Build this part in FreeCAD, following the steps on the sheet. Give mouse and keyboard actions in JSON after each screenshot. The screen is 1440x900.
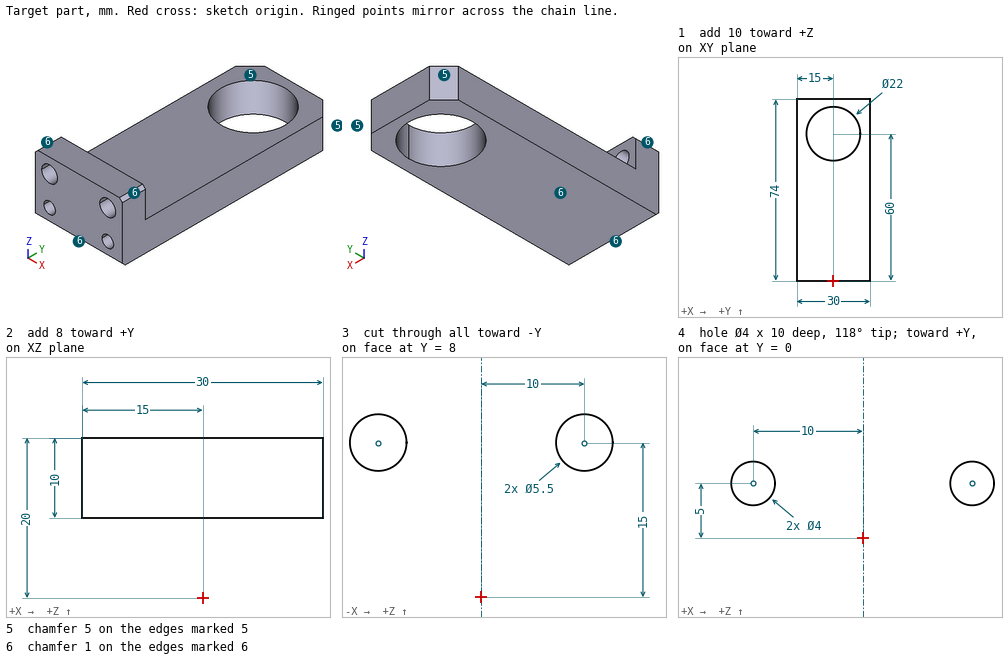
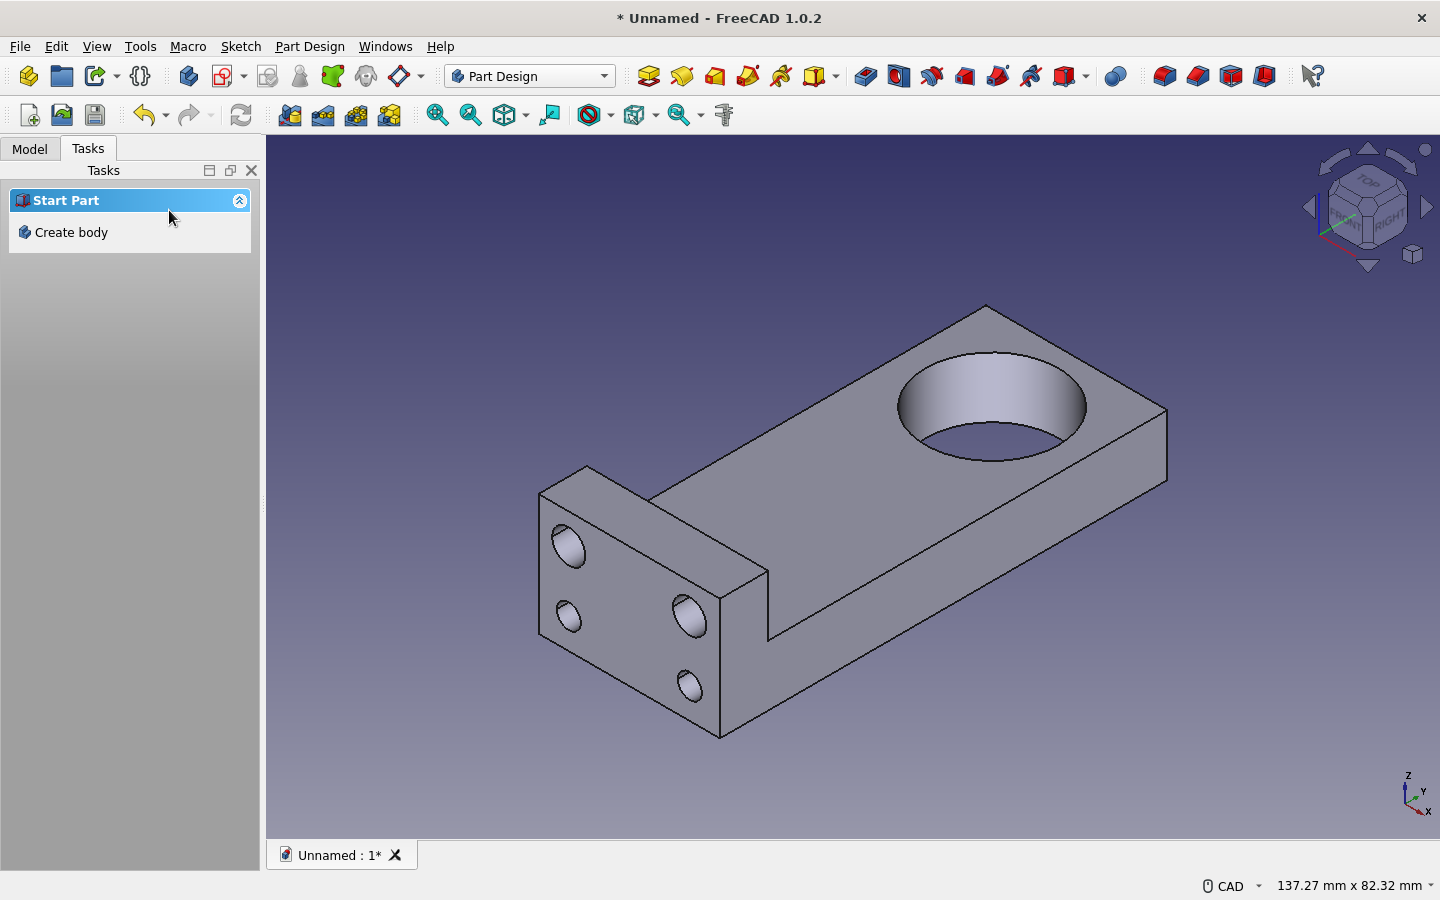
{"action": "key", "text": "1"}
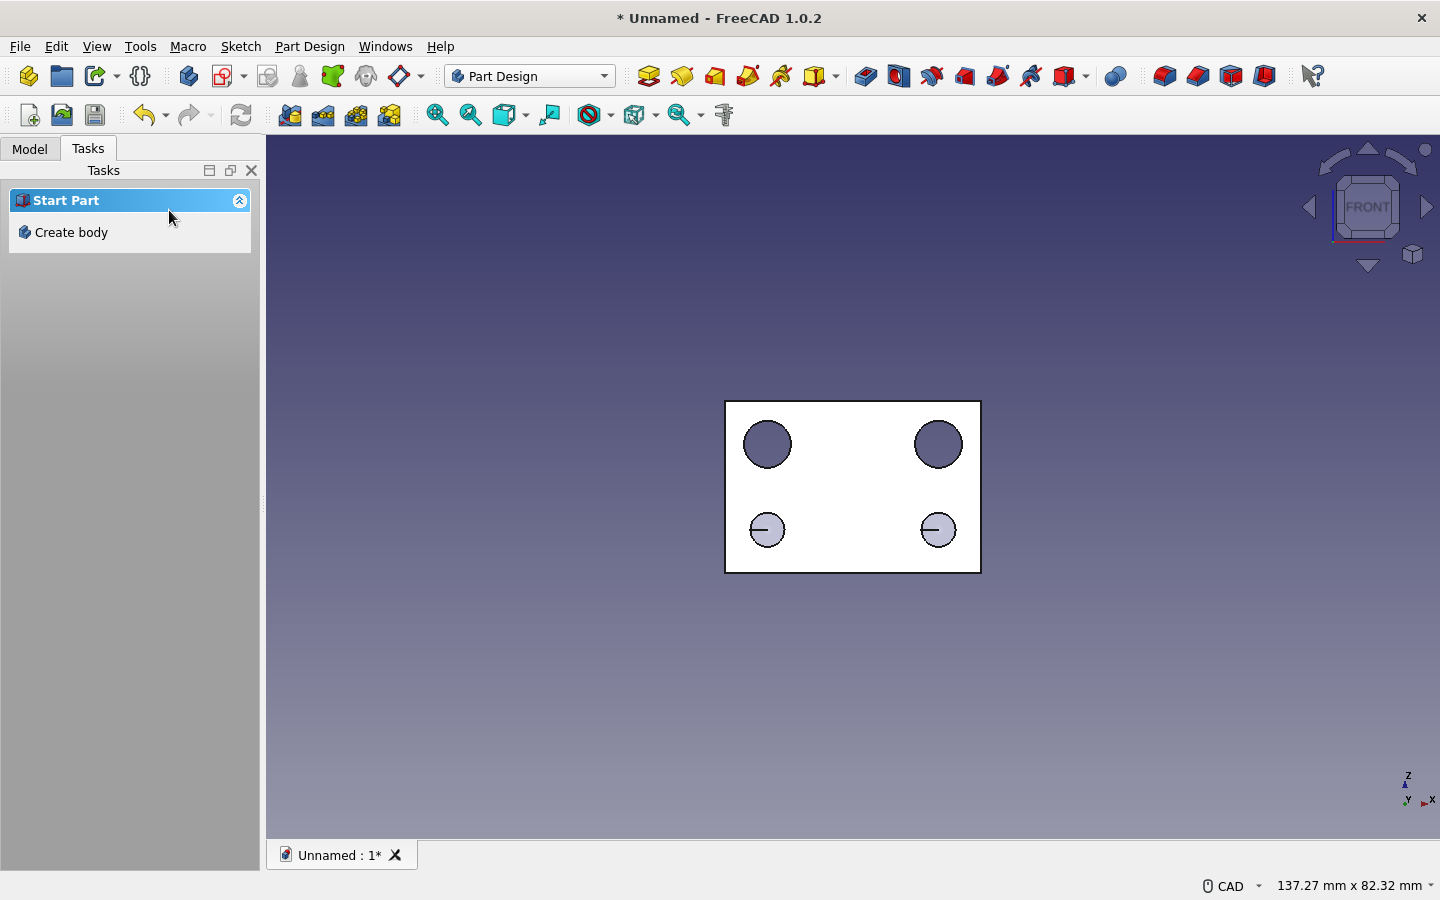
{"action": "left_click", "coordinate": [438, 116]}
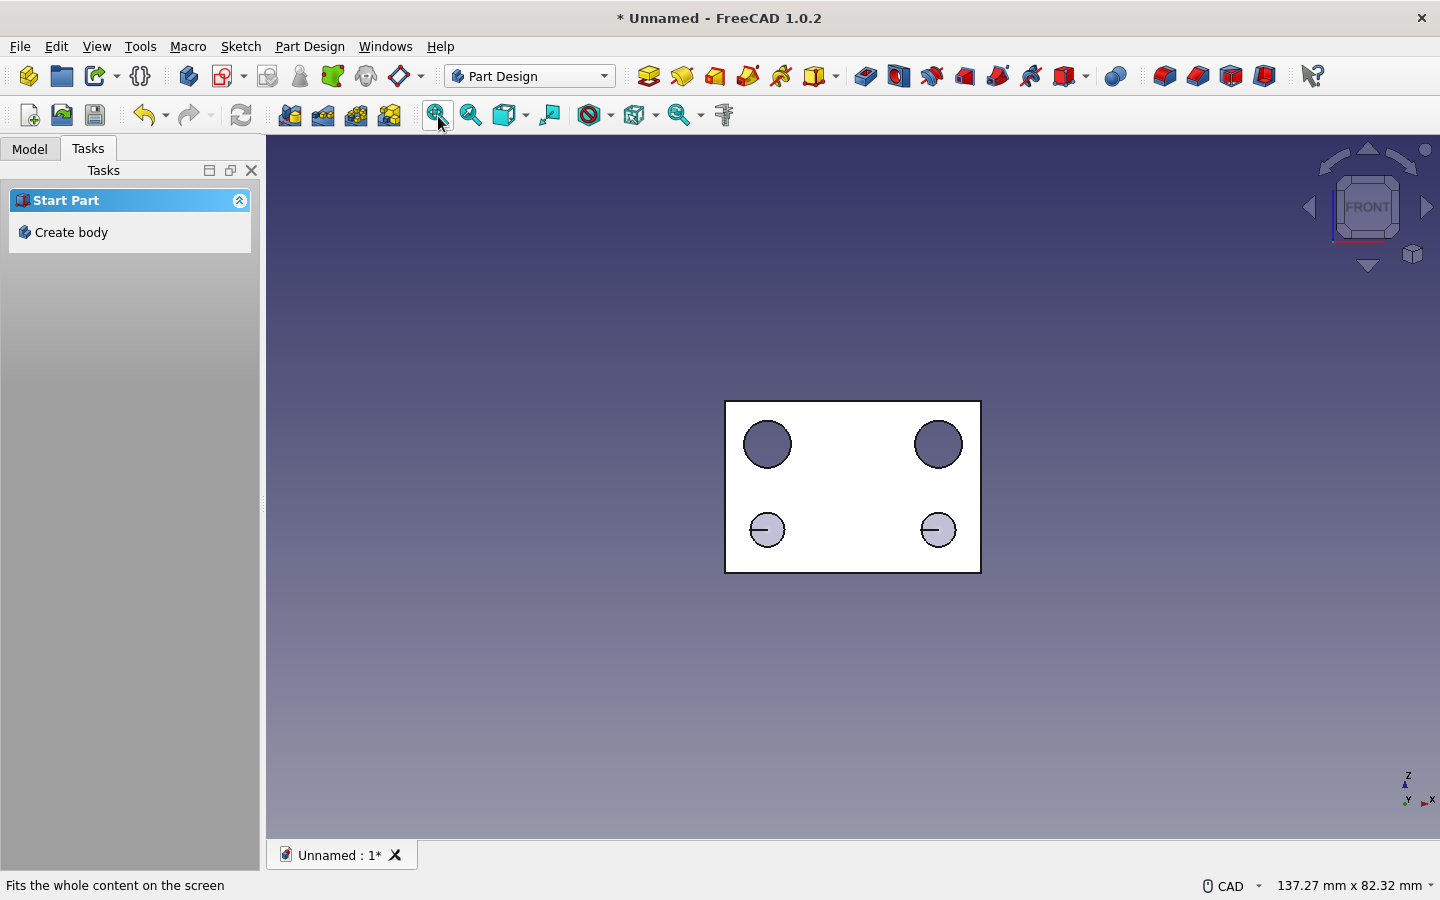
{"action": "key", "text": "3"}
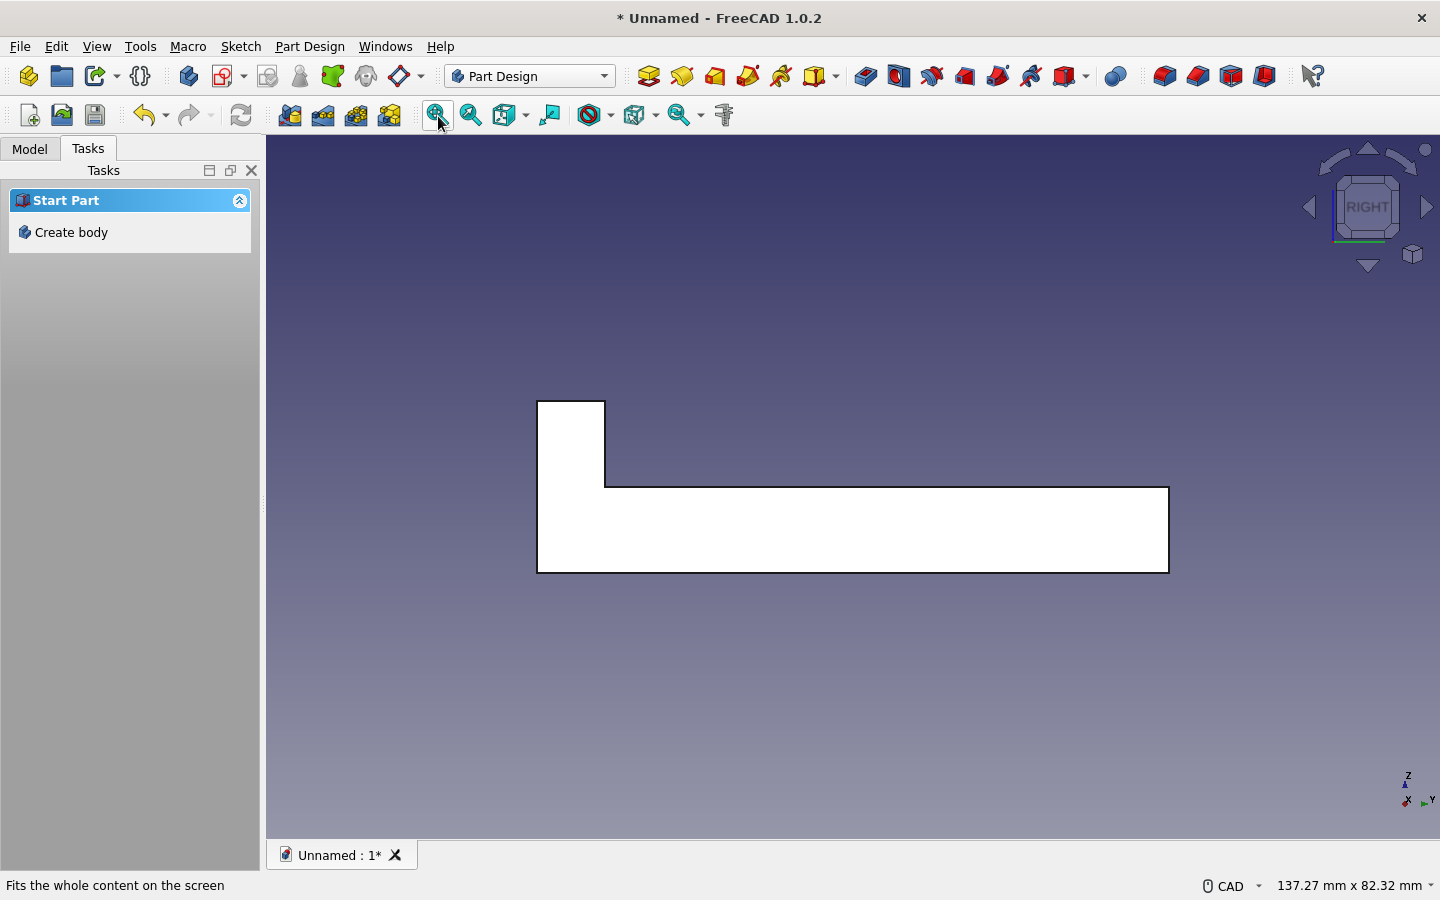
{"action": "left_click", "coordinate": [1169, 529]}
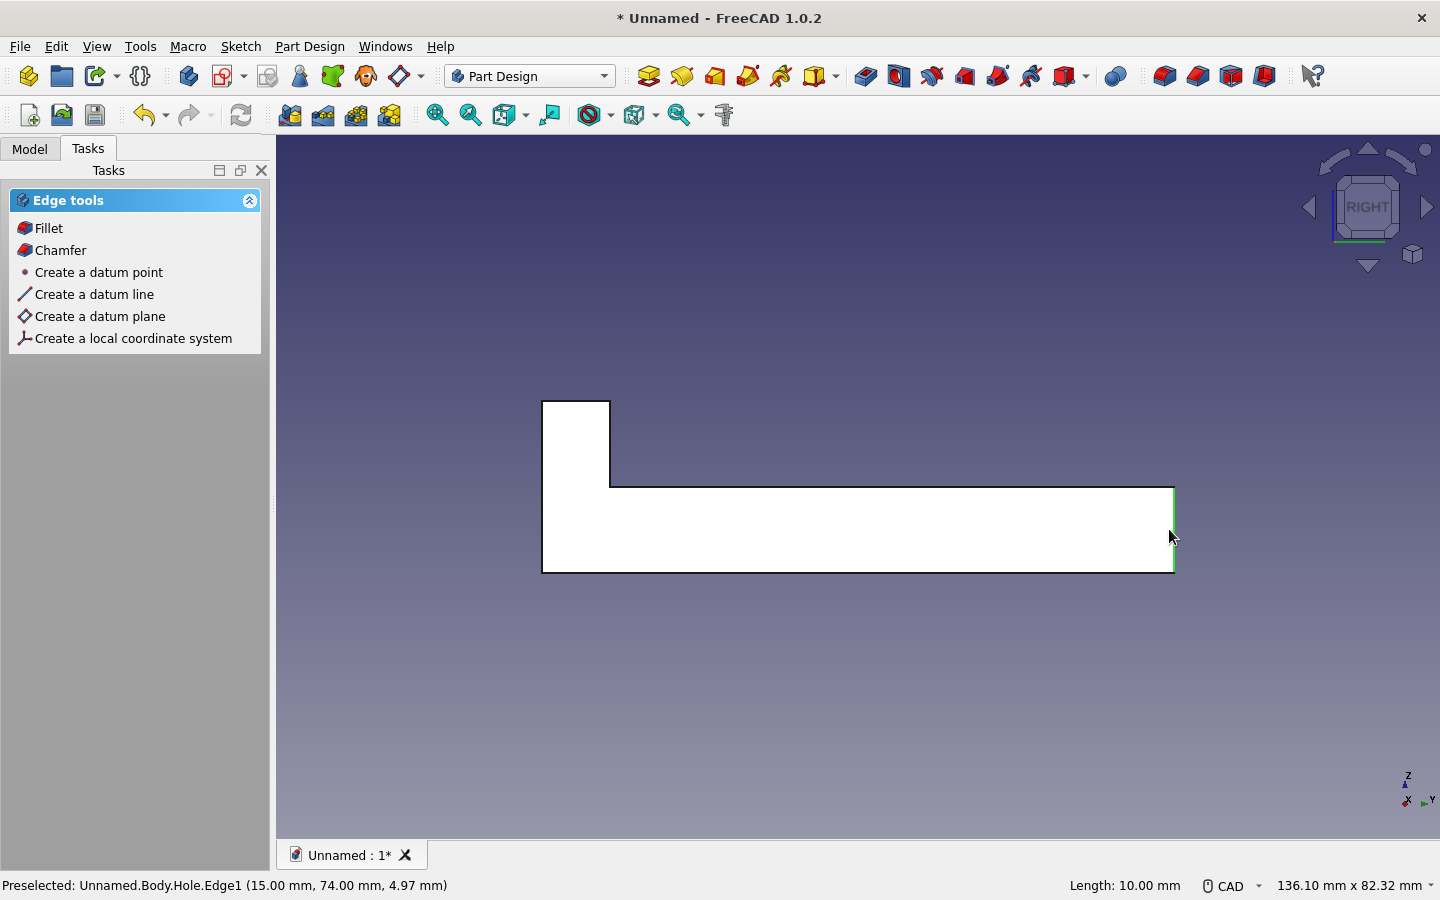
{"action": "key", "text": "5"}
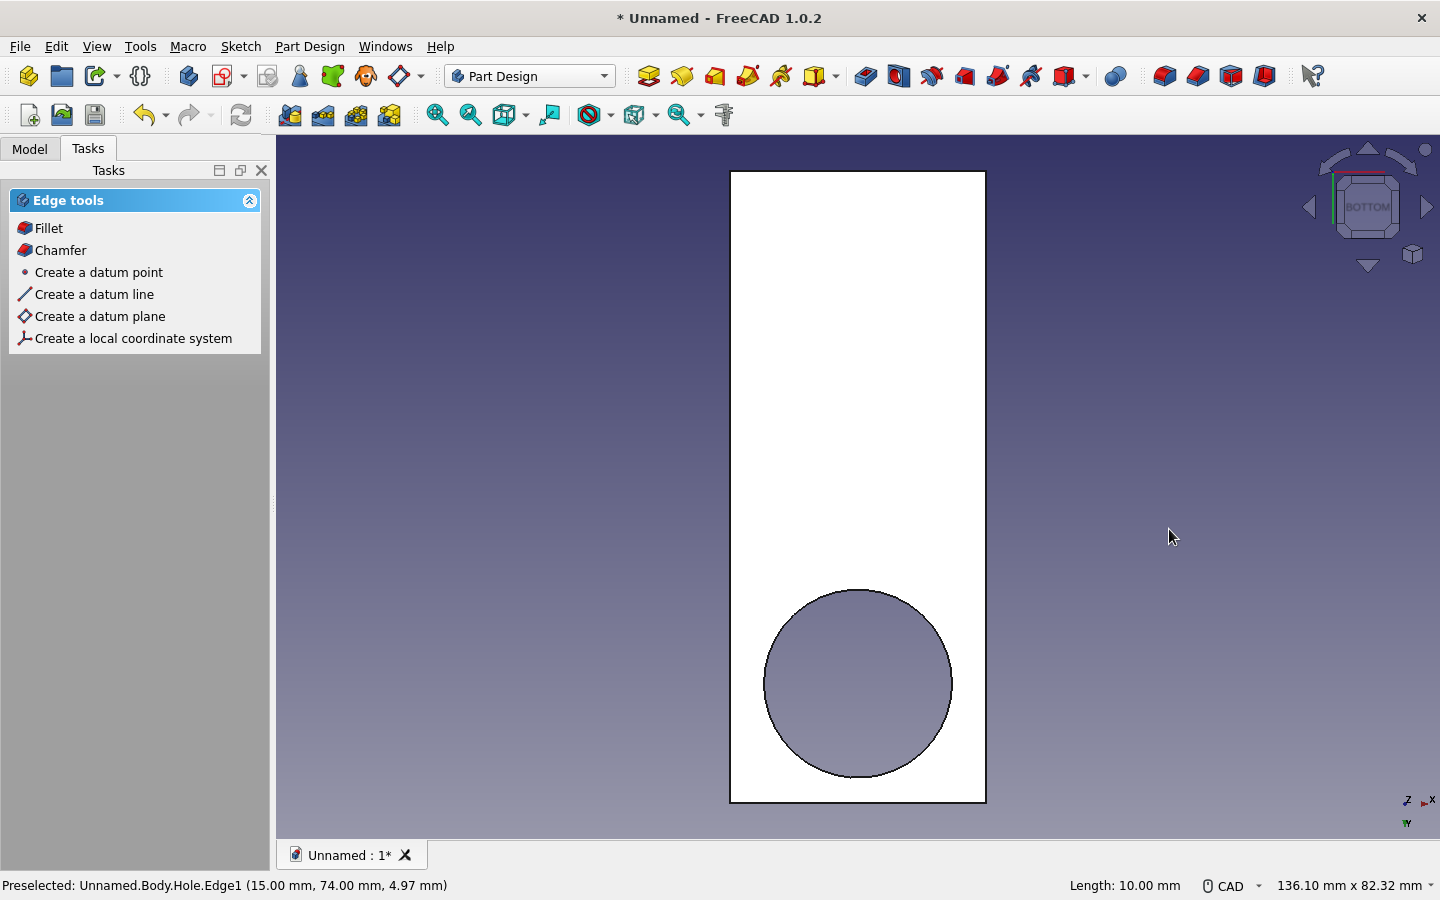
{"action": "key", "text": "4"}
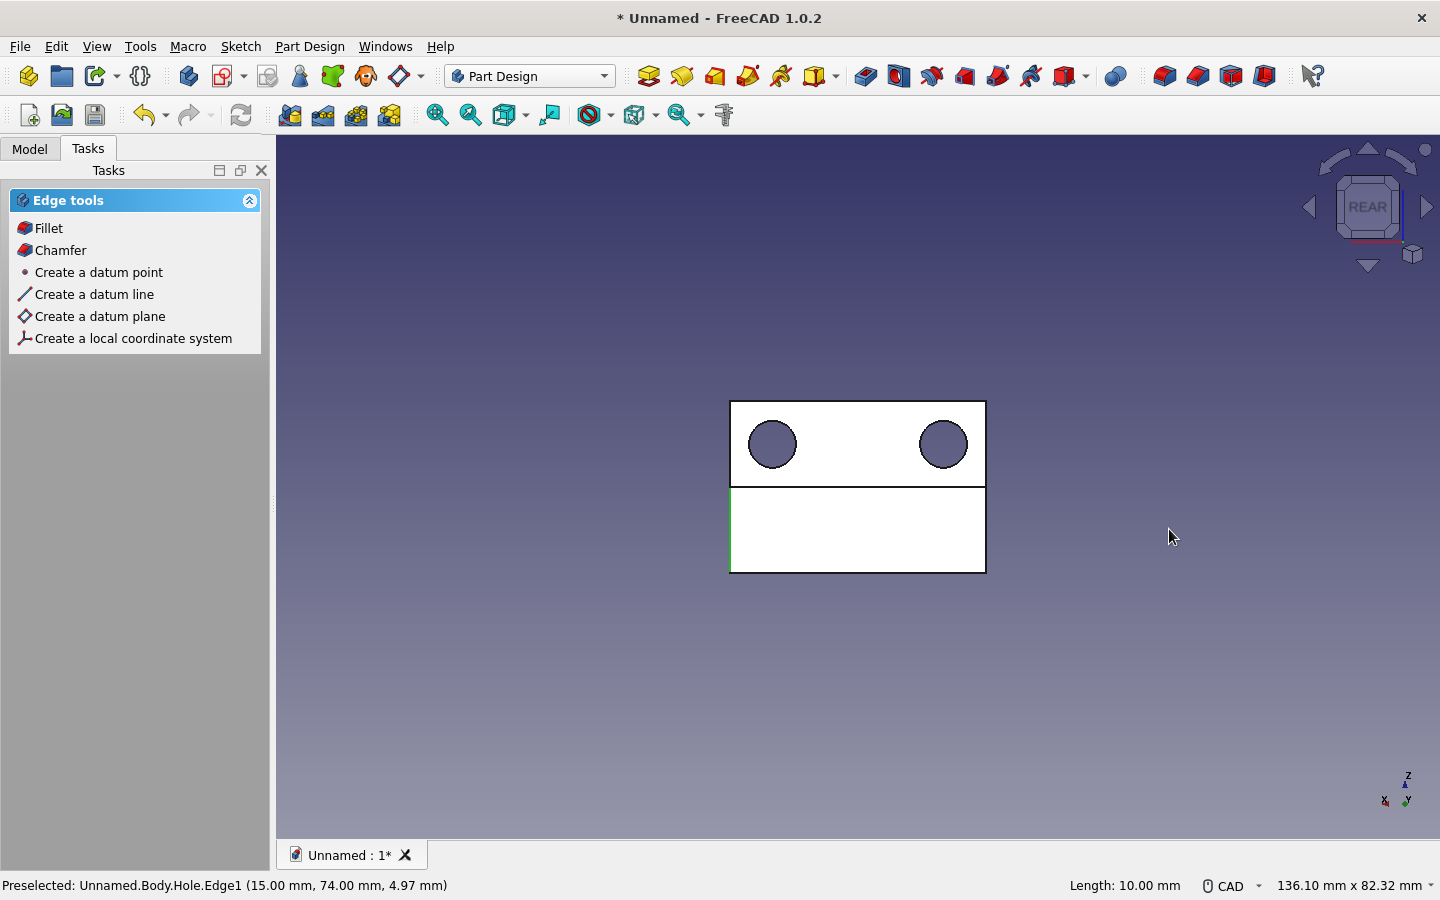
{"action": "left_click", "coordinate": [438, 116]}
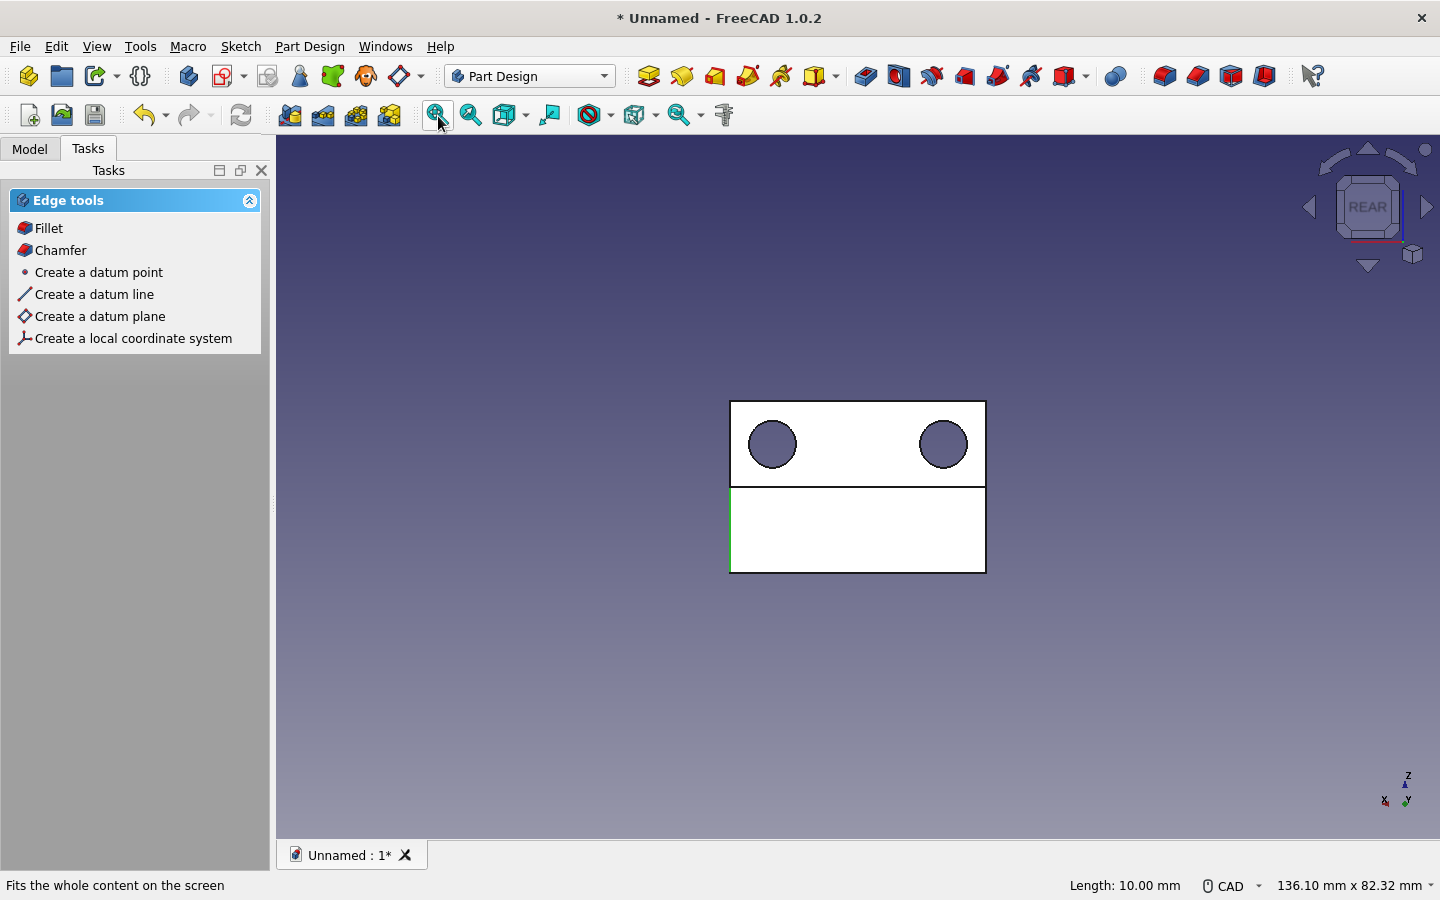
{"action": "left_click", "coordinate": [986, 529], "text": "ctrl"}